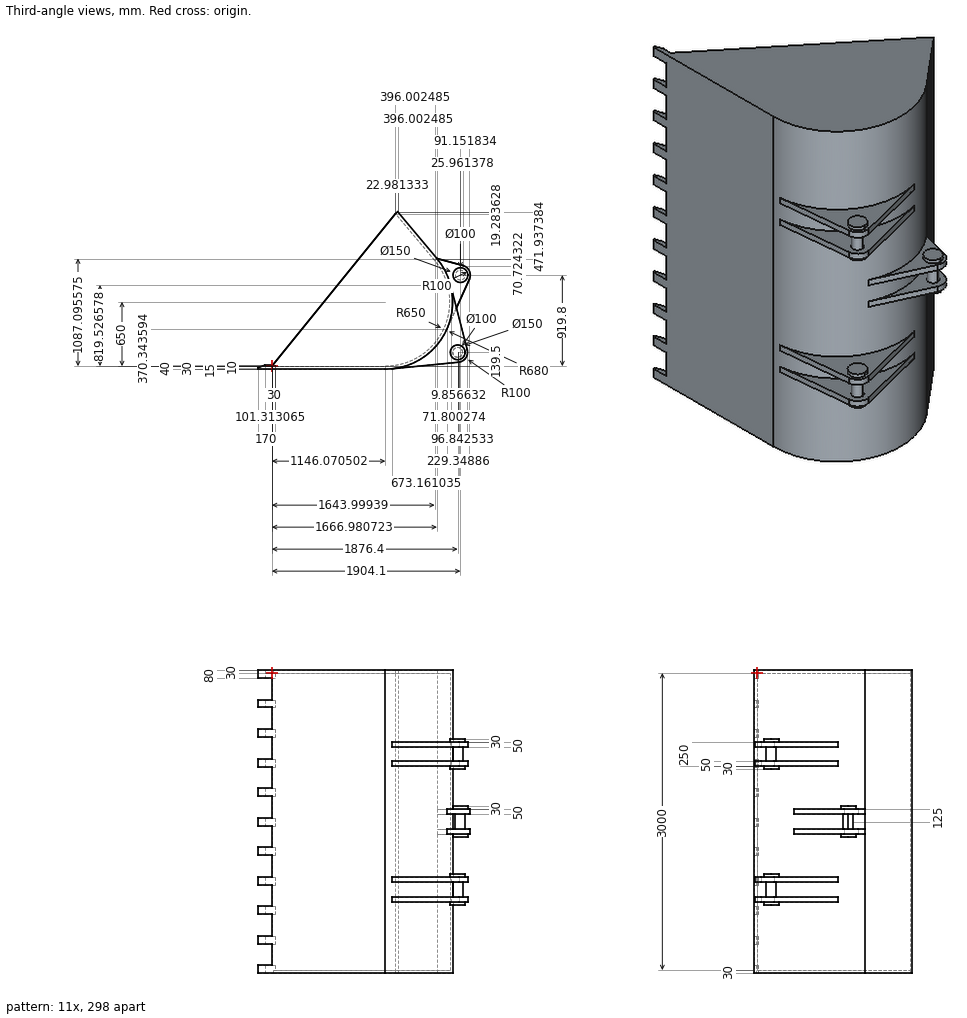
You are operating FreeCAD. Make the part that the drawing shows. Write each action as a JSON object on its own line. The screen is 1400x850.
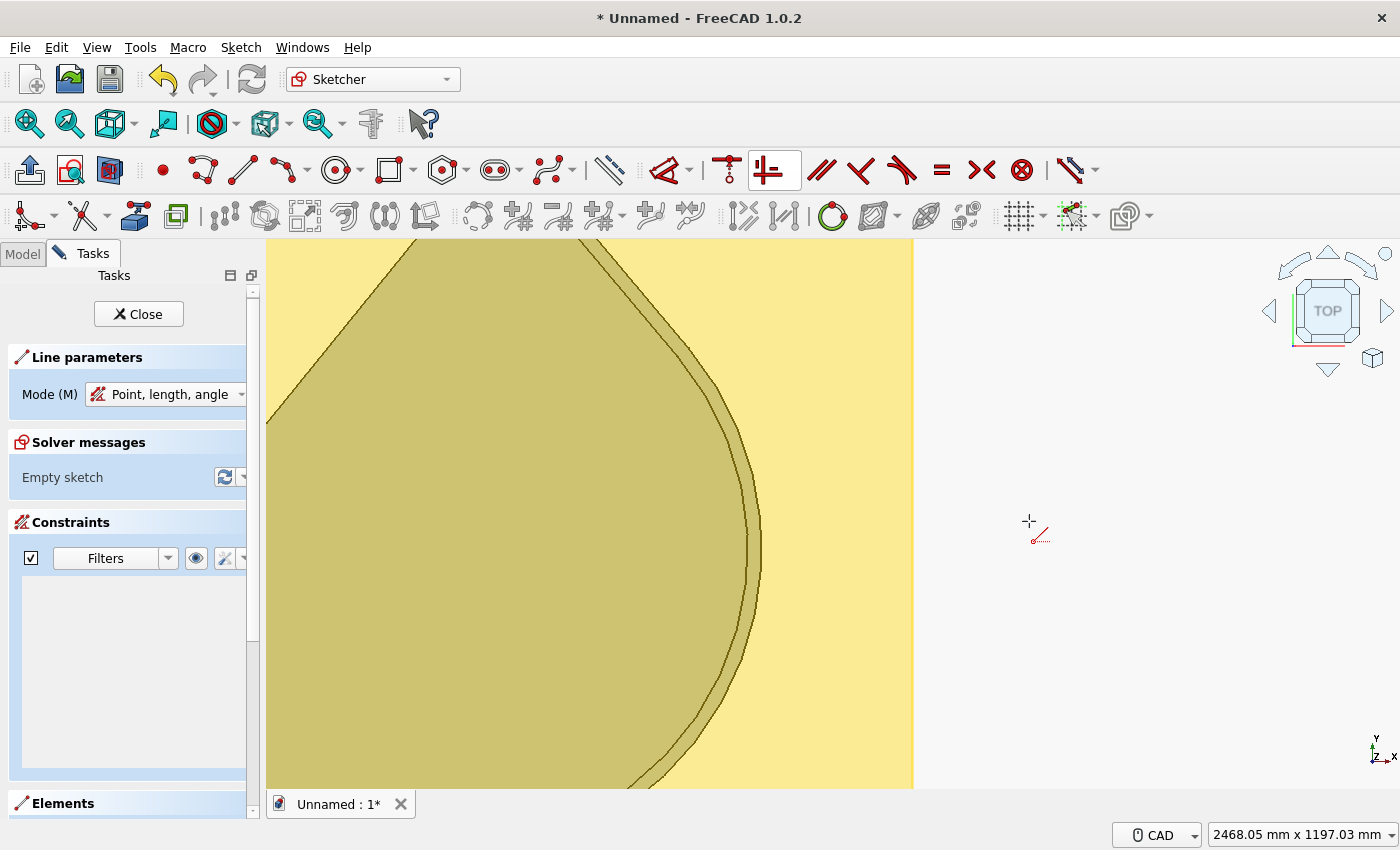
{"action": "left_click", "coordinate": [809, 381]}
{"action": "left_click", "coordinate": [689, 348]}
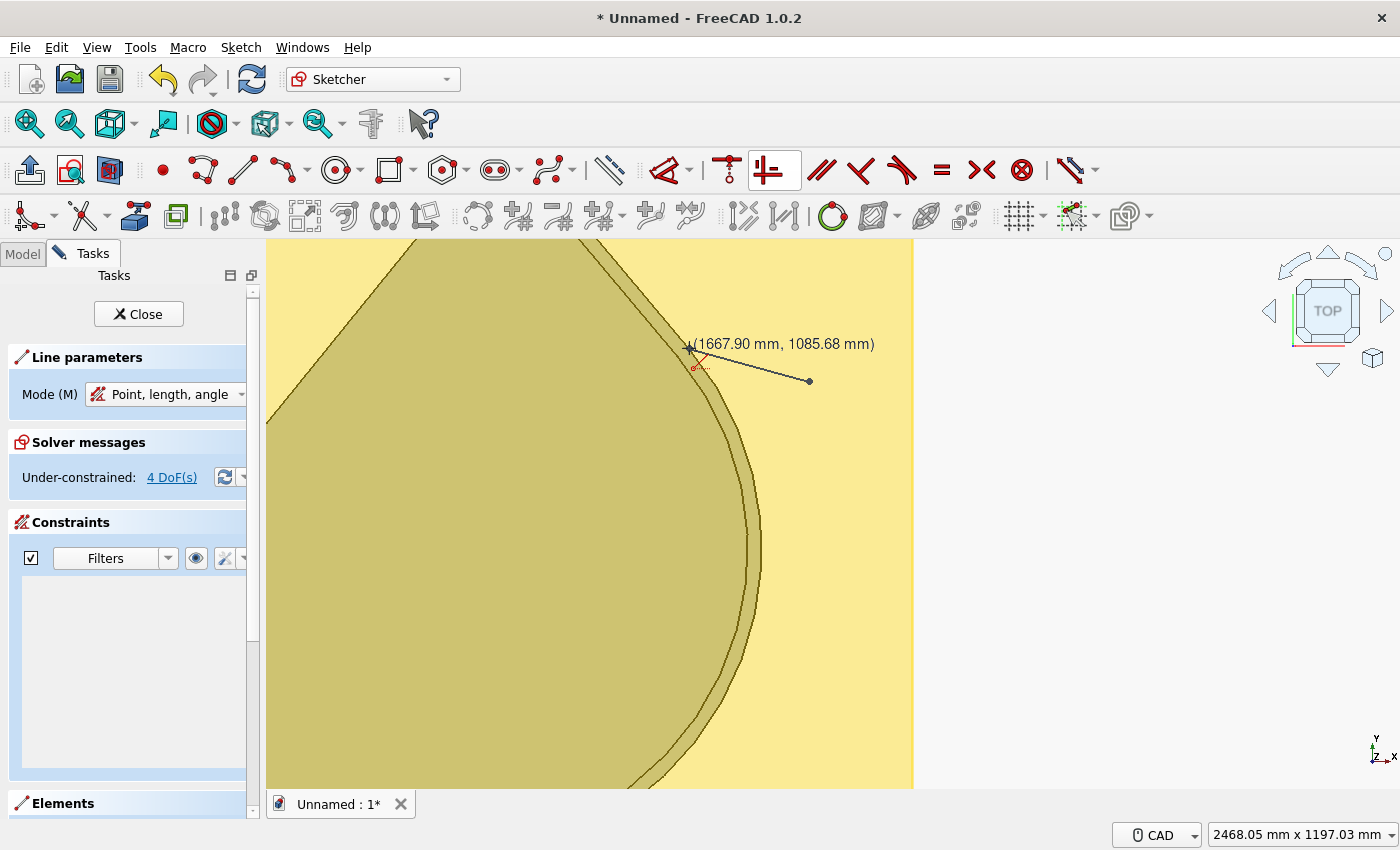
{"action": "left_click", "coordinate": [734, 678]}
{"action": "left_click", "coordinate": [839, 444]}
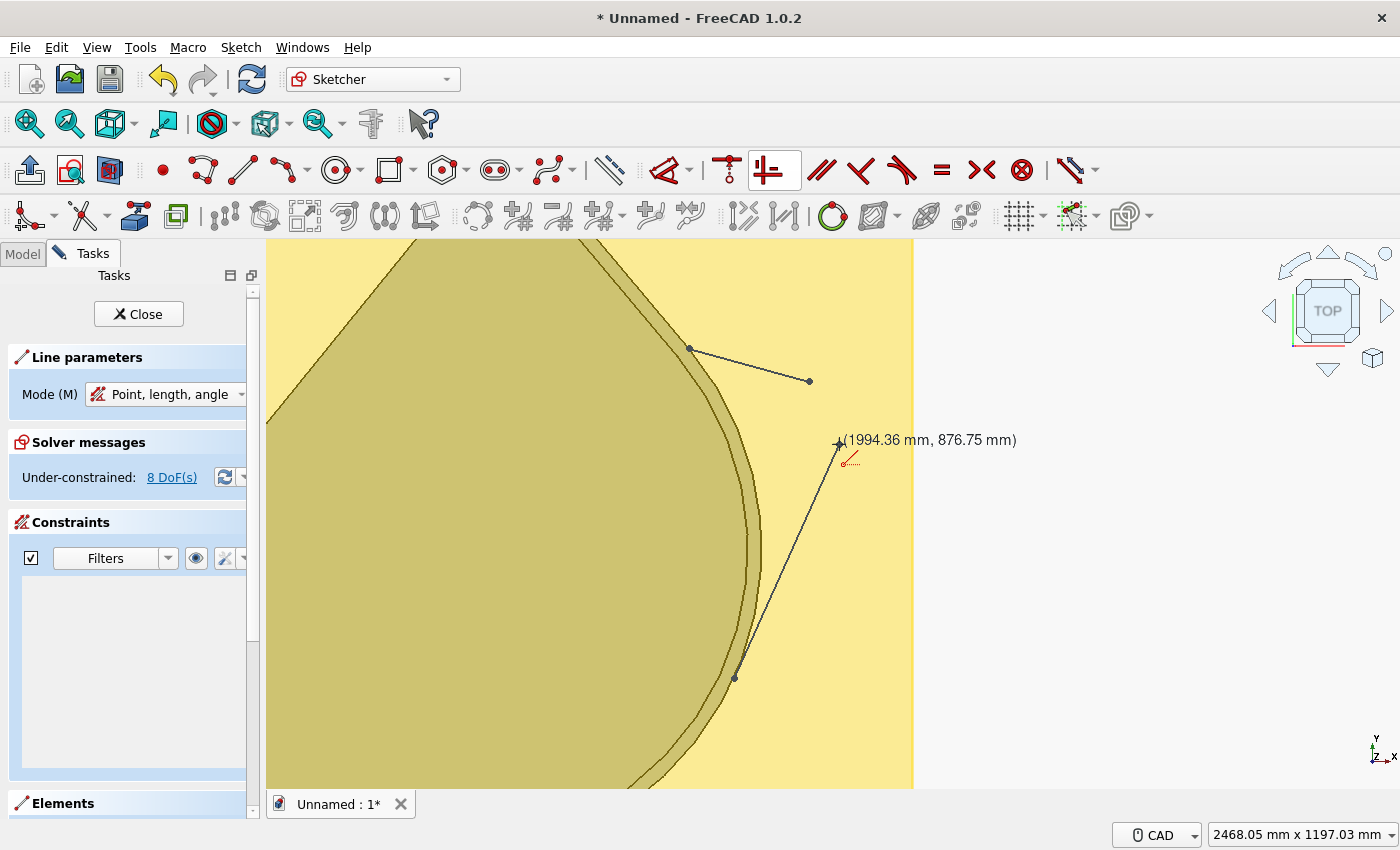
{"action": "left_click", "coordinate": [284, 170]}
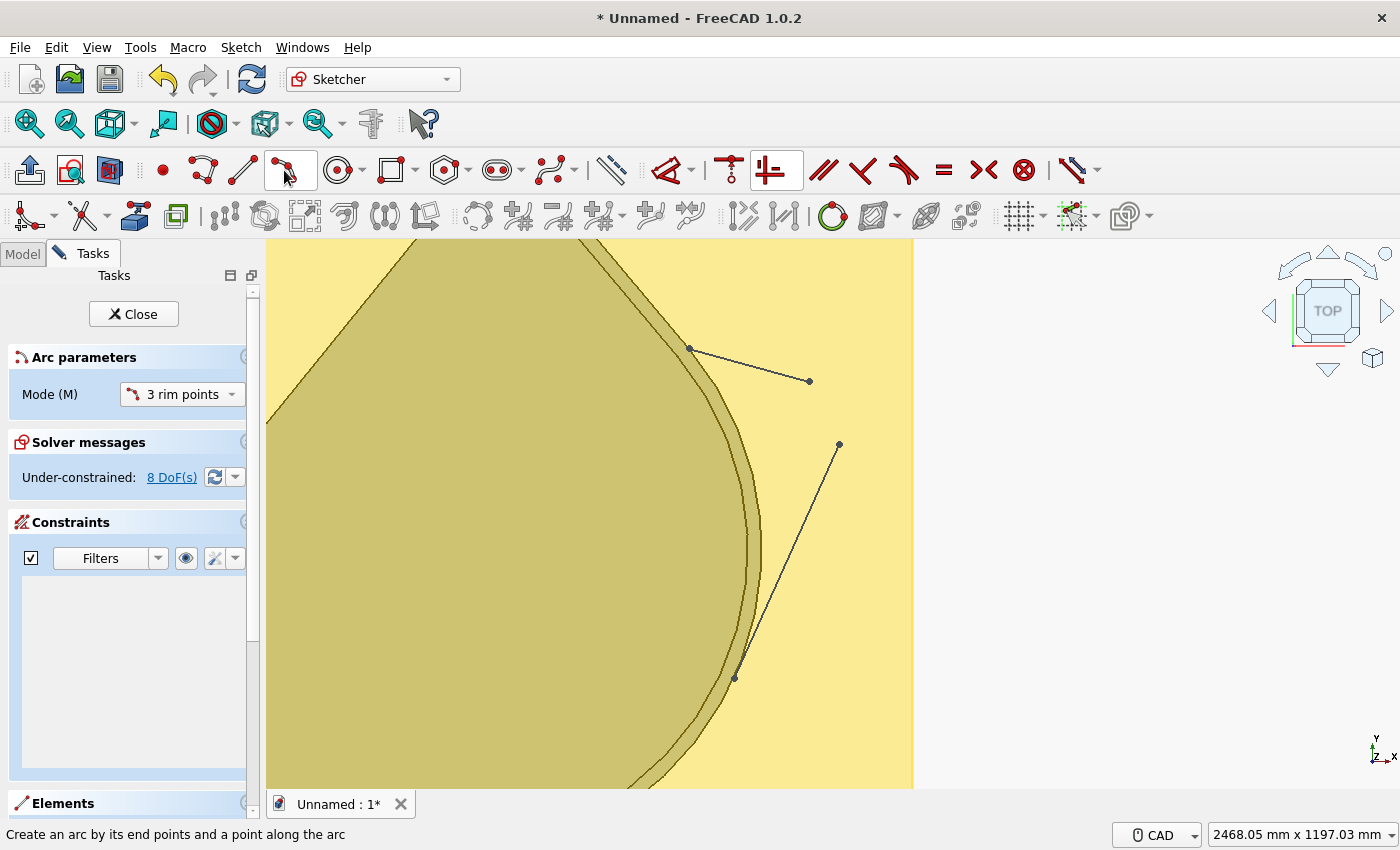
{"action": "left_click", "coordinate": [689, 349]}
{"action": "left_click", "coordinate": [734, 679]}
{"action": "left_click", "coordinate": [759, 506]}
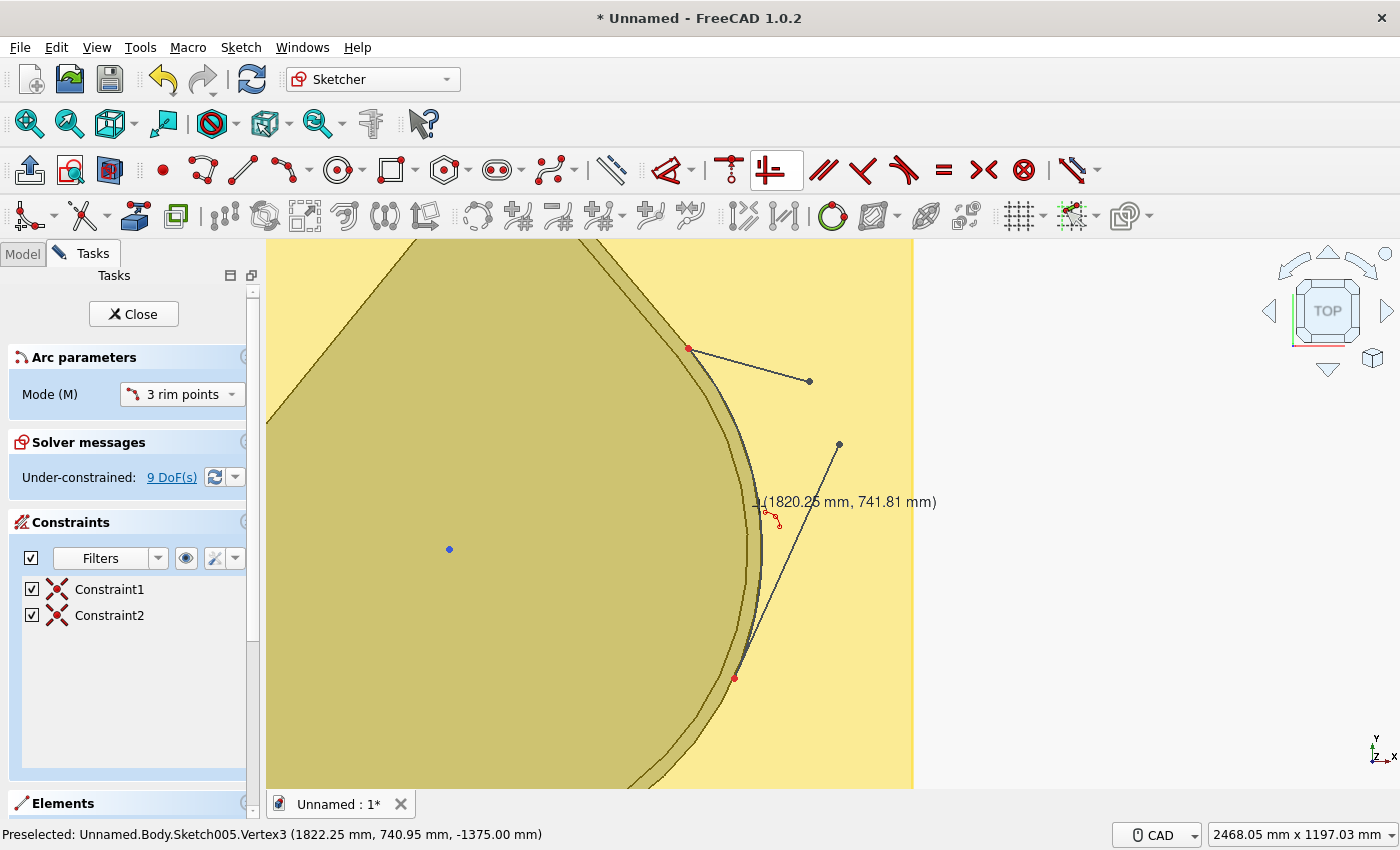
{"action": "left_click", "coordinate": [839, 445]}
{"action": "left_click", "coordinate": [809, 382]}
{"action": "left_click", "coordinate": [839, 406]}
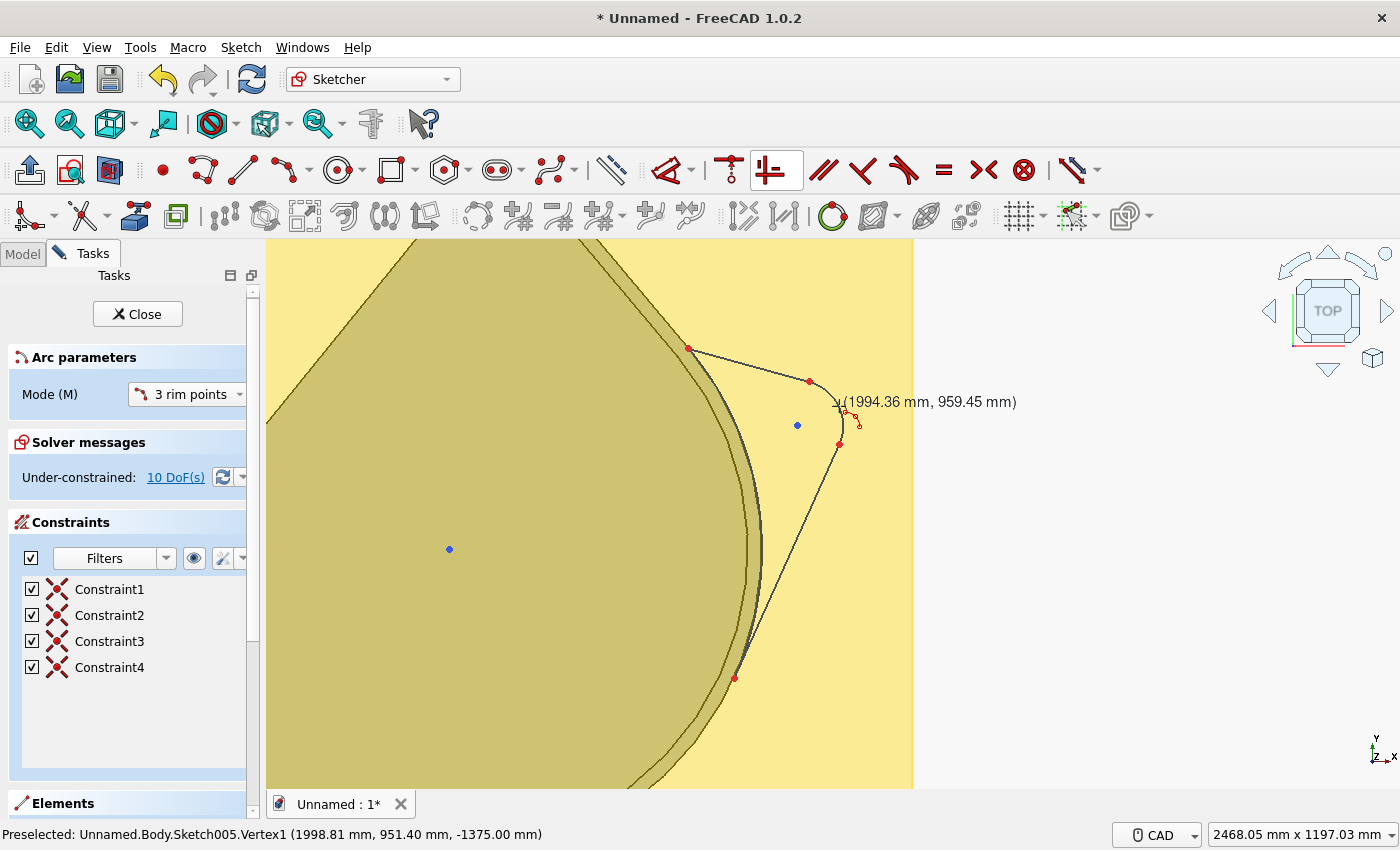
{"action": "left_click", "coordinate": [338, 170]}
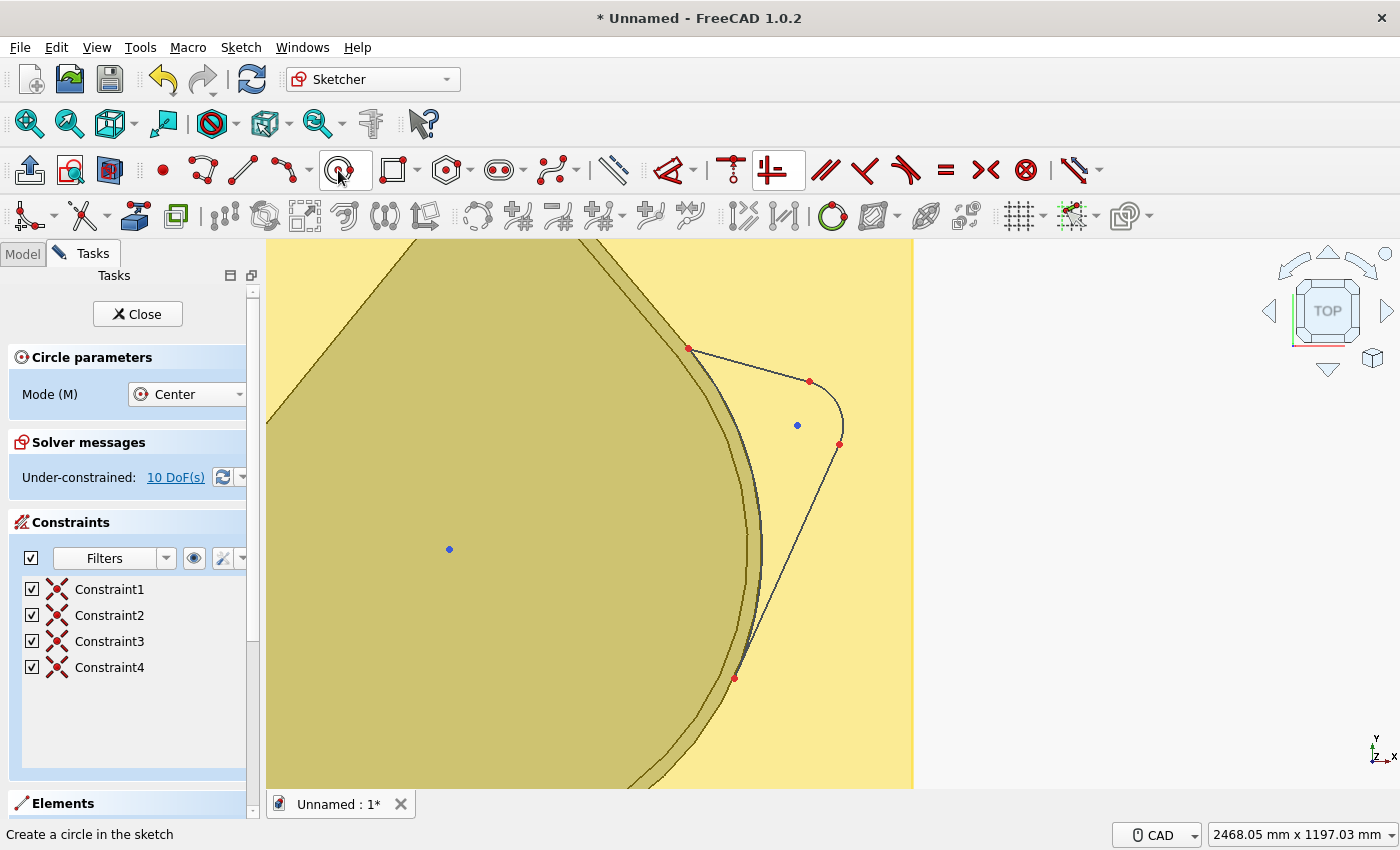
{"action": "left_click", "coordinate": [798, 425]}
{"action": "left_click", "coordinate": [814, 409]}
{"action": "key", "text": "Escape"}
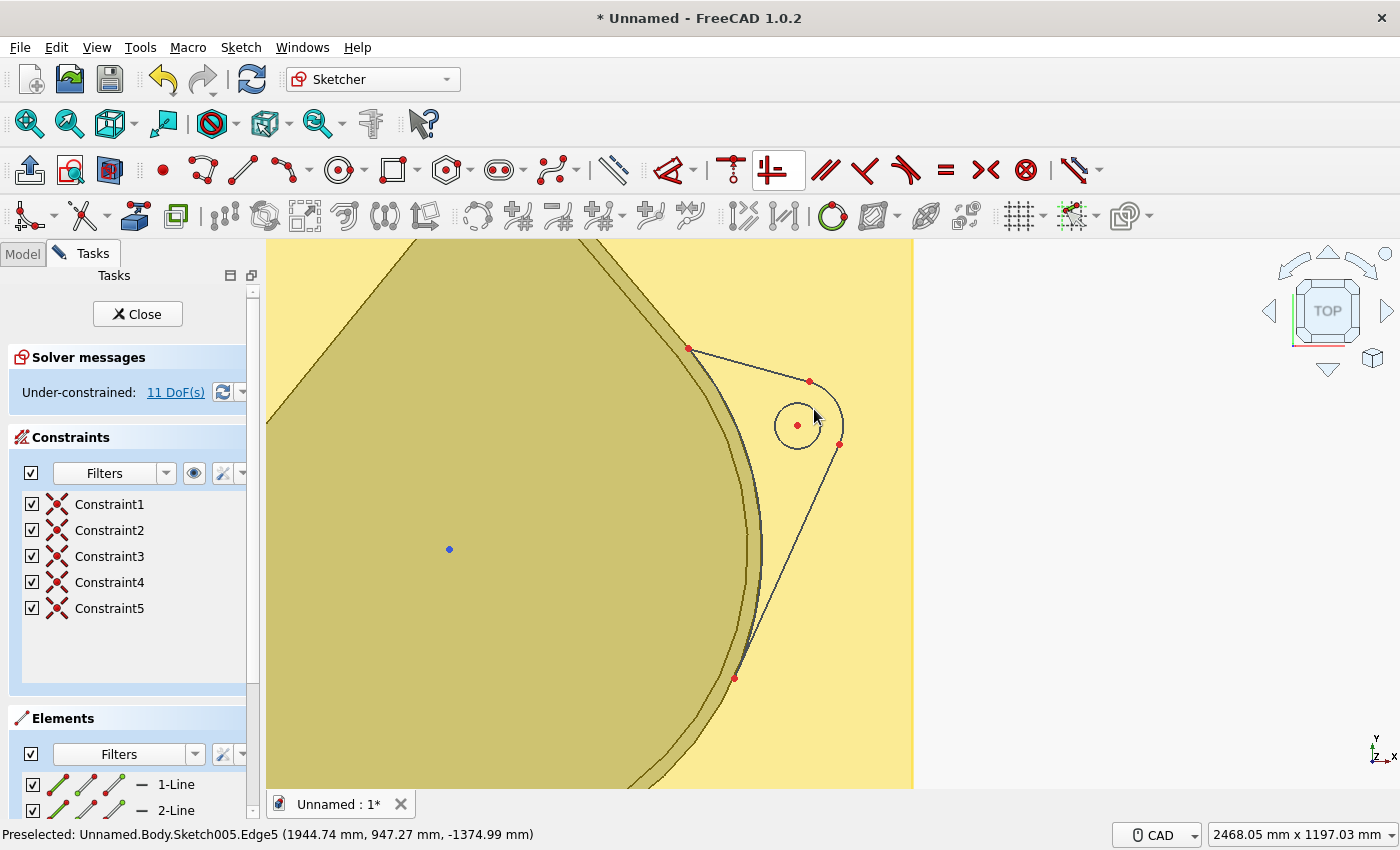
{"action": "key", "text": "d"}